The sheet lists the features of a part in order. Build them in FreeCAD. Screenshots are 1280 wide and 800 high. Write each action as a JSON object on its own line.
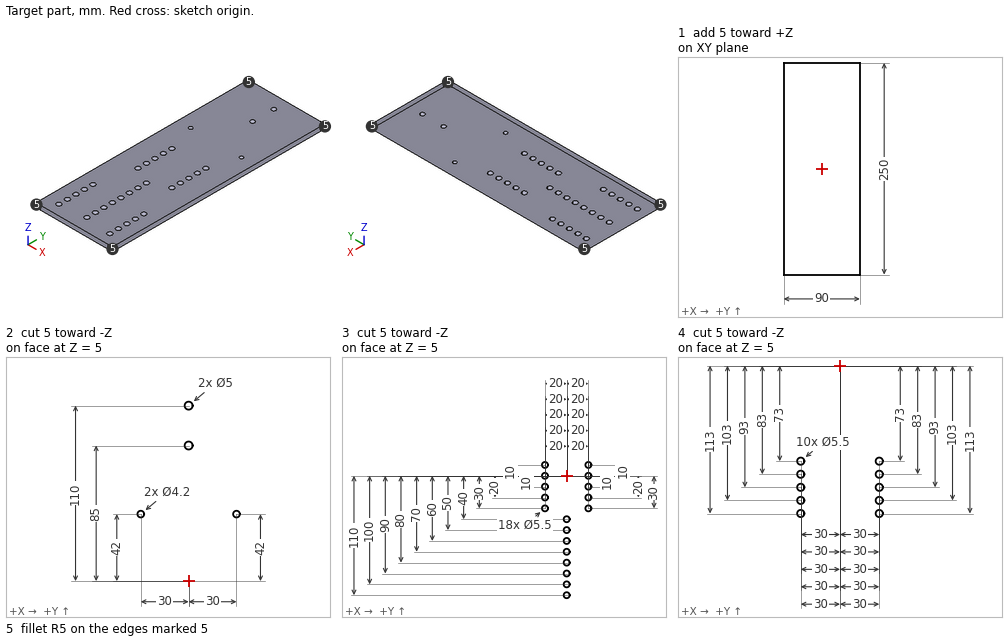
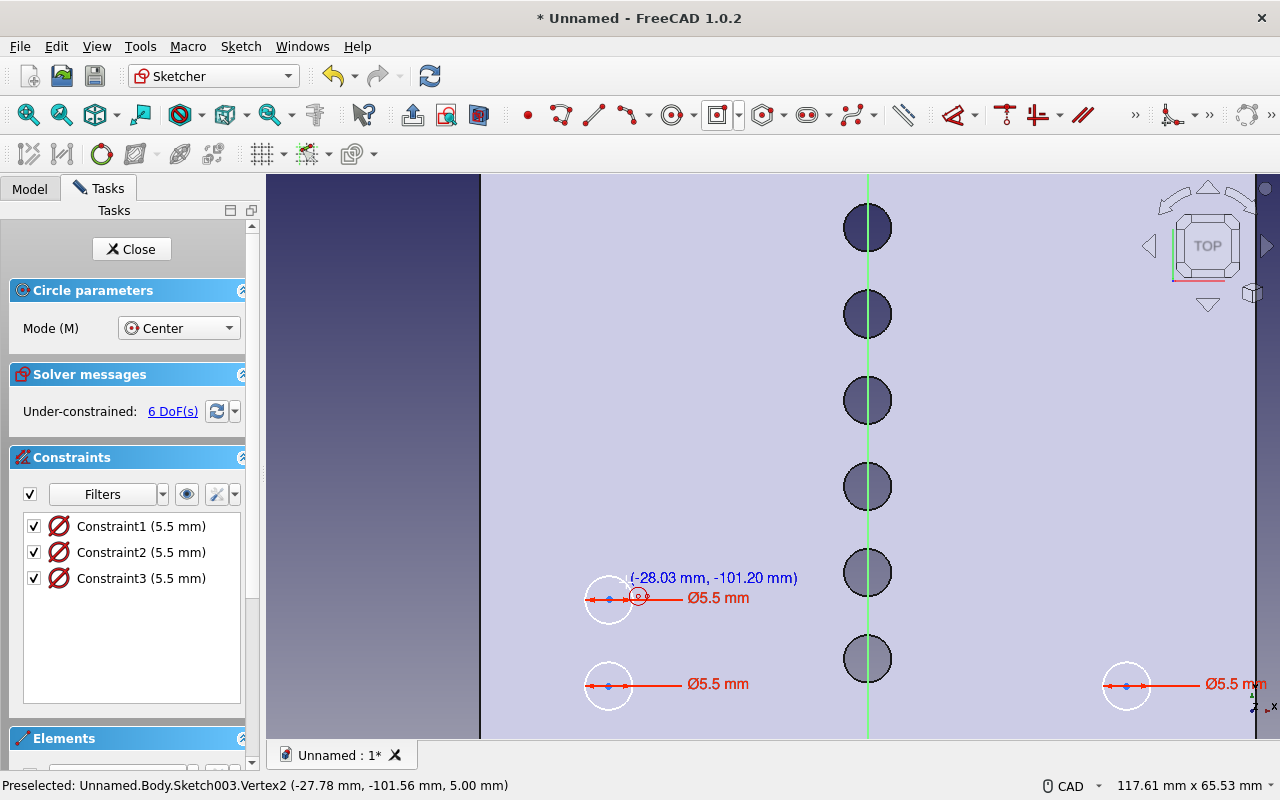
{"action": "scroll", "coordinate": [610, 600], "scroll_direction": "down", "scroll_amount": 5}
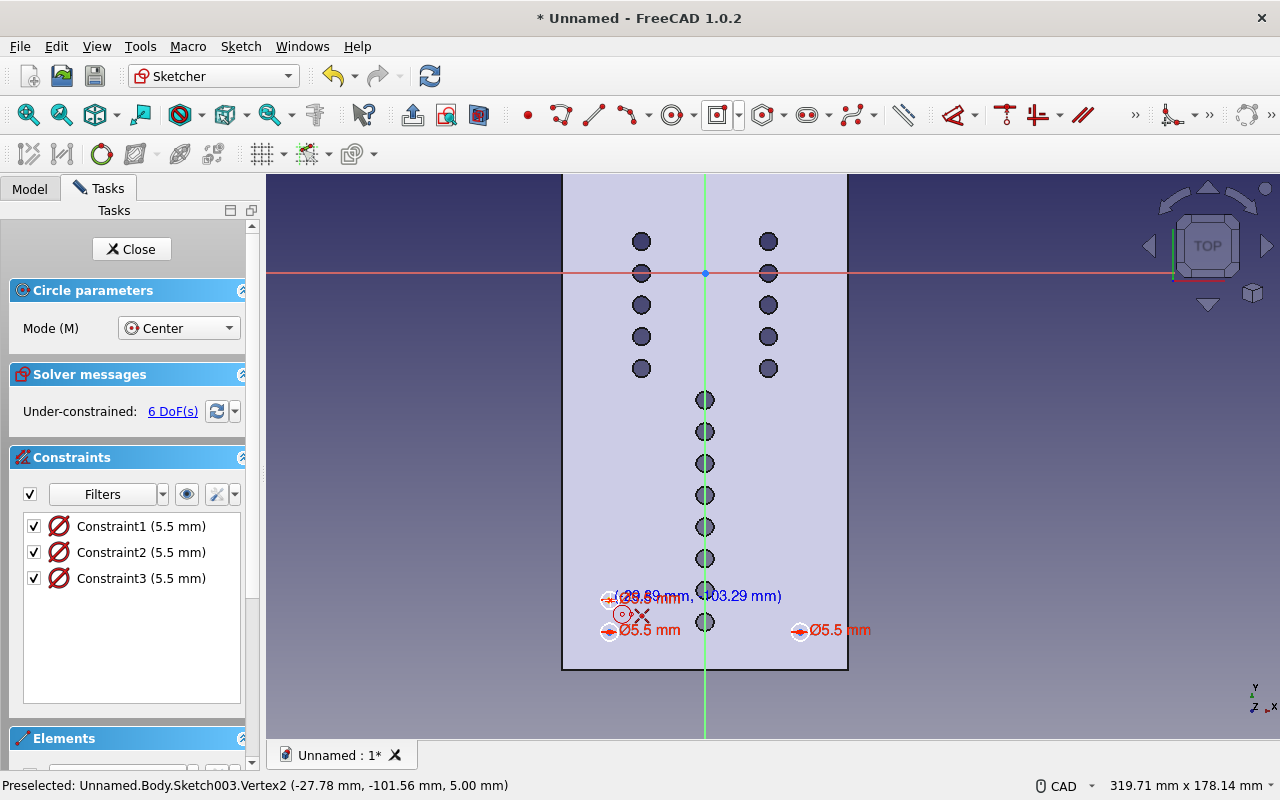
{"action": "scroll", "coordinate": [800, 600], "scroll_direction": "up", "scroll_amount": 5}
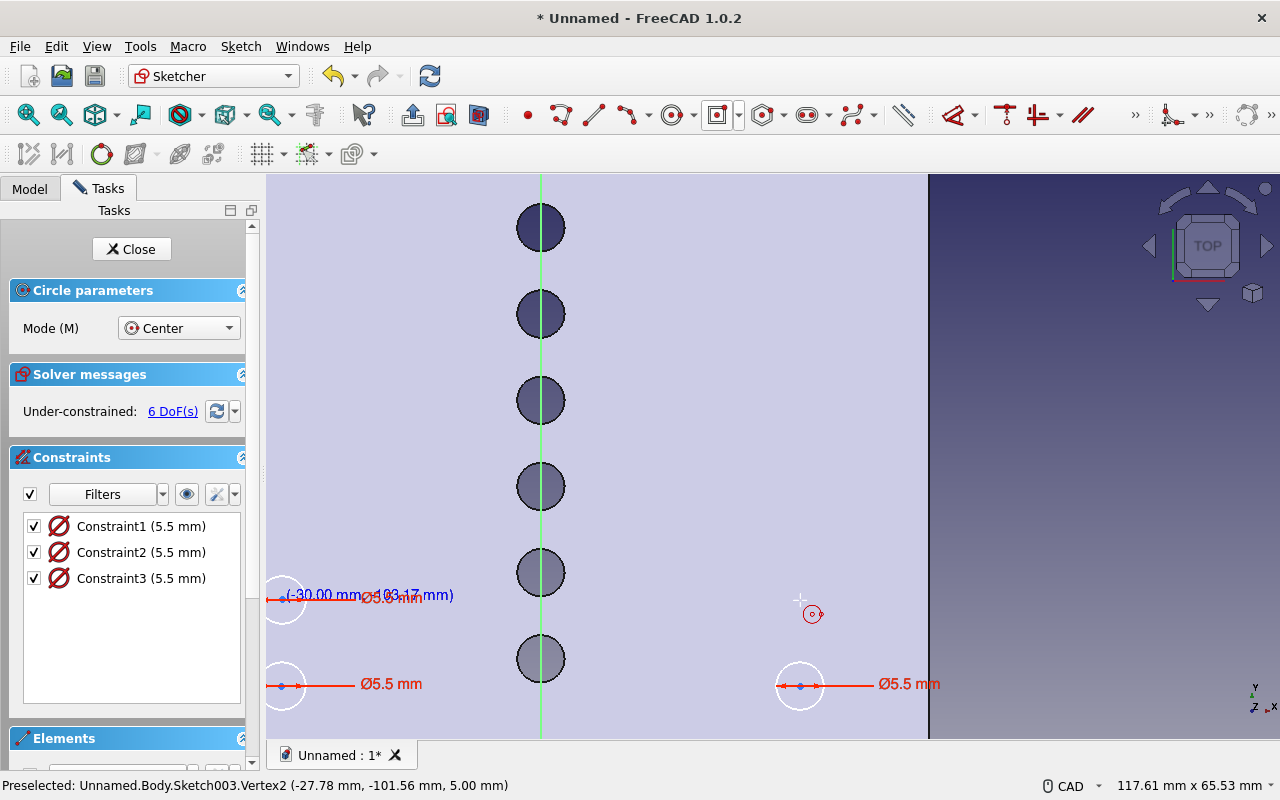
{"action": "left_click", "coordinate": [800, 599]}
{"action": "mouse_move", "coordinate": [816, 582]}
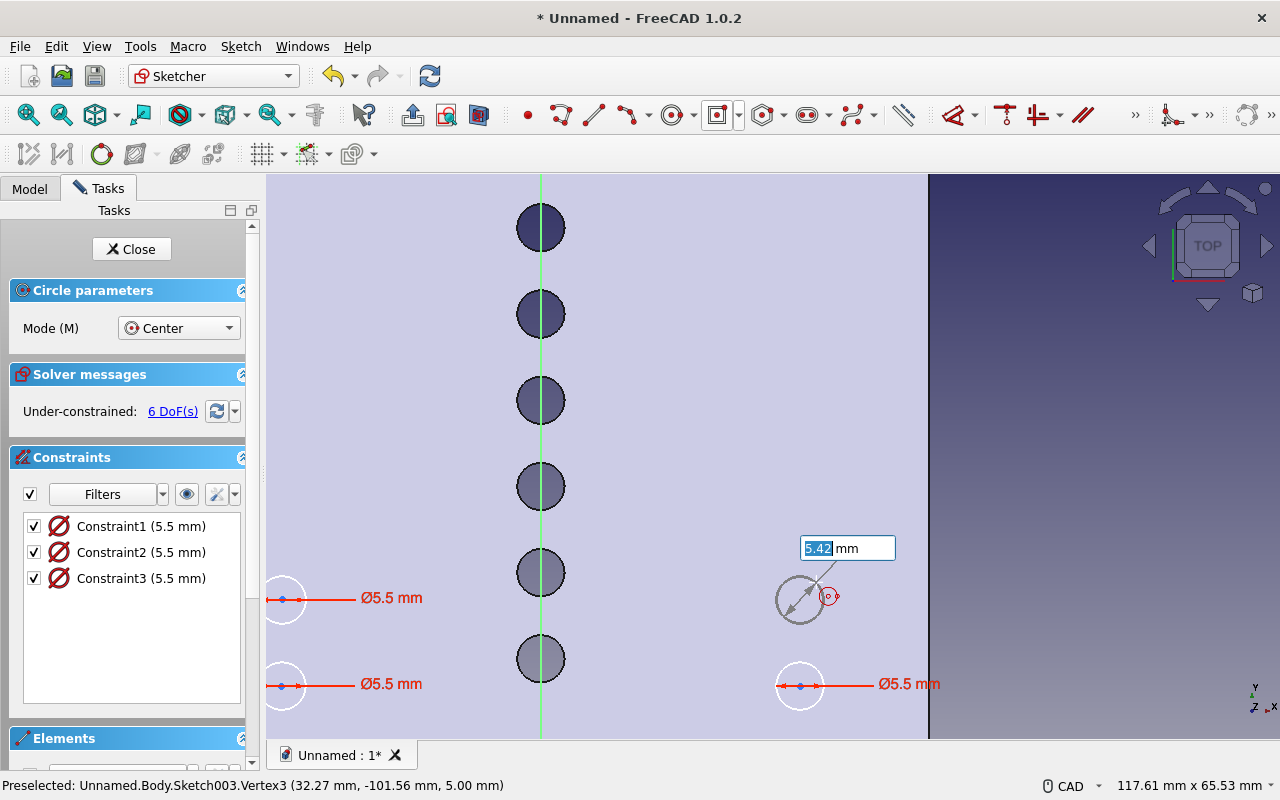
{"action": "type", "text": "5.5"}
{"action": "key", "text": "Return"}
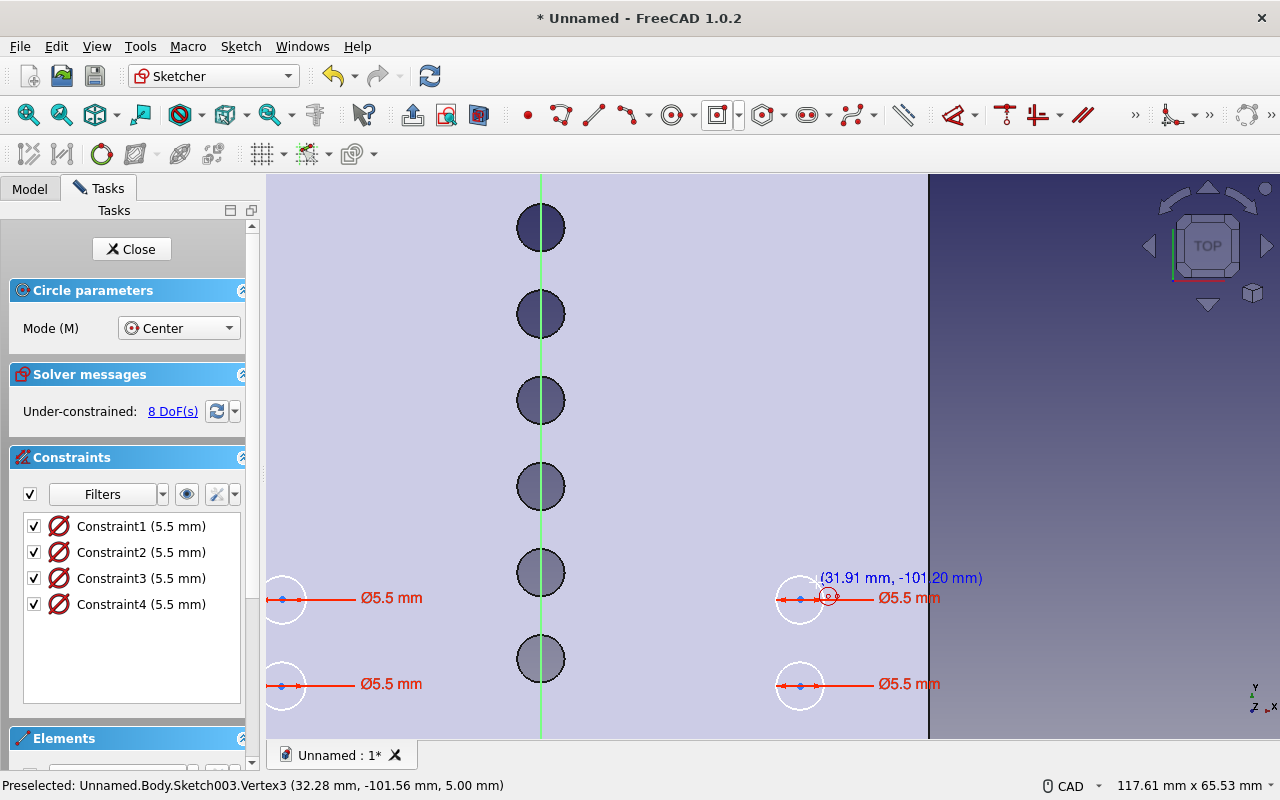
{"action": "scroll", "coordinate": [800, 600], "scroll_direction": "down", "scroll_amount": 5}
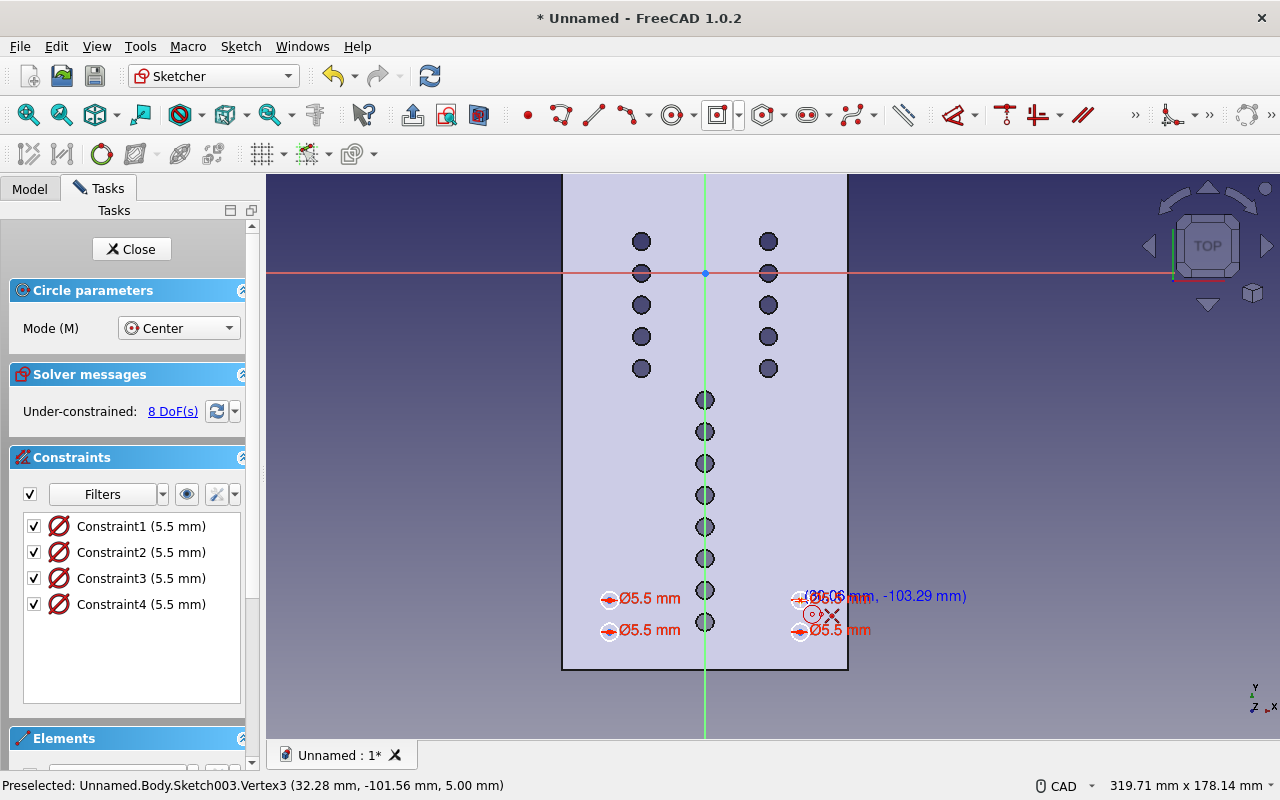
{"action": "scroll", "coordinate": [610, 568], "scroll_direction": "up", "scroll_amount": 5}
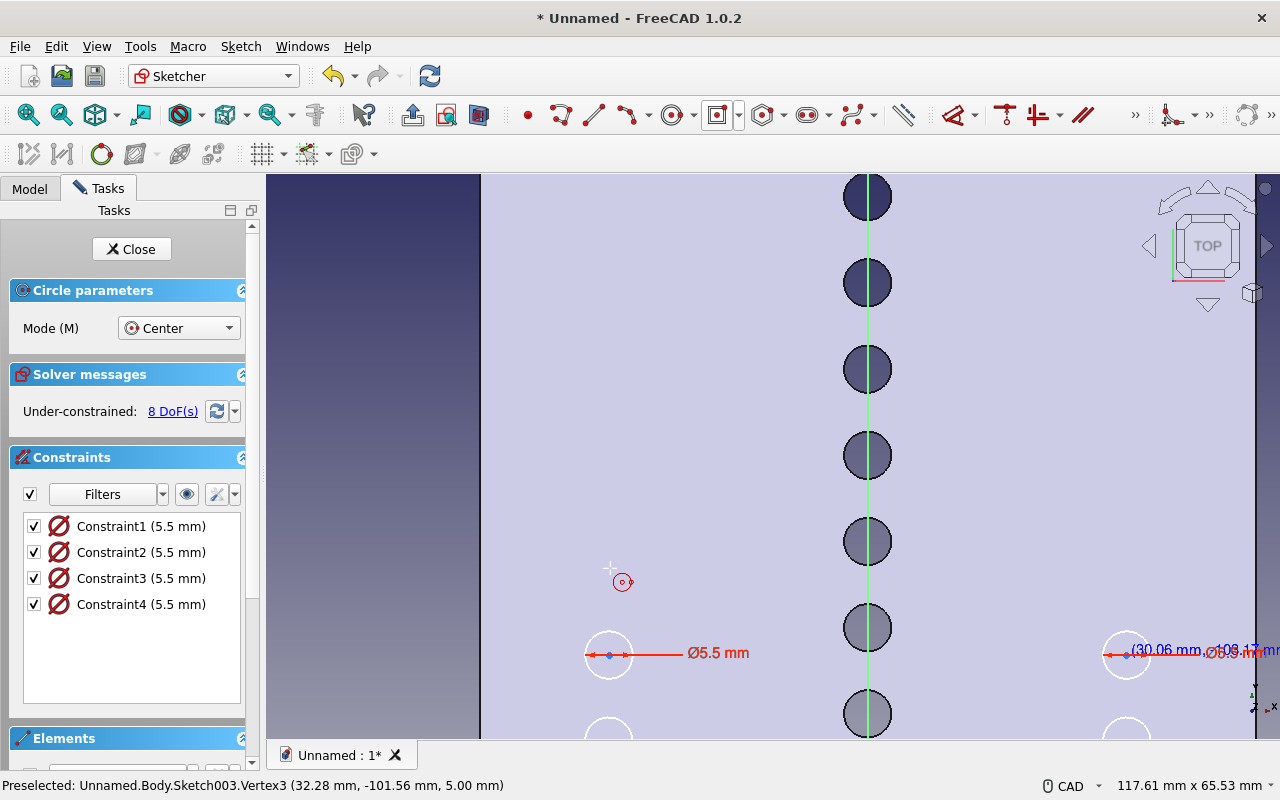
{"action": "left_click", "coordinate": [609, 567]}
{"action": "mouse_move", "coordinate": [626, 551]}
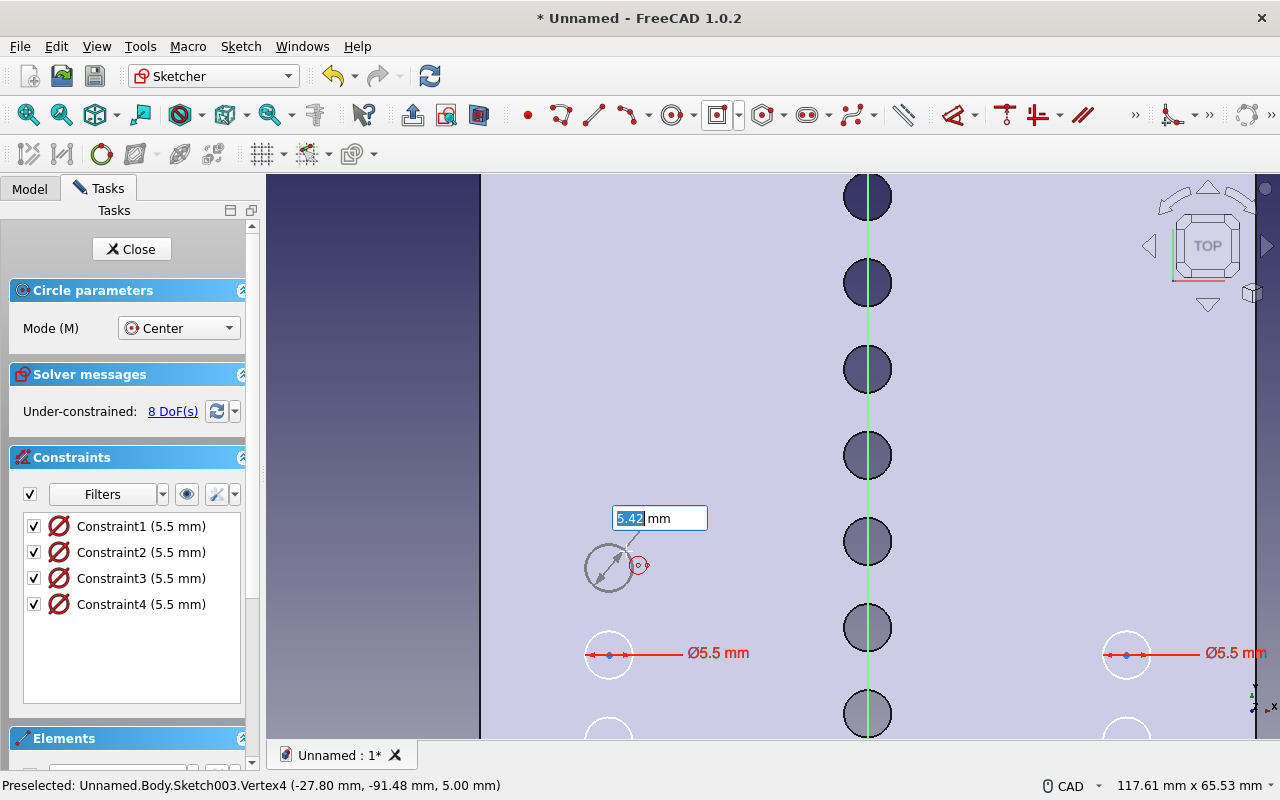
{"action": "type", "text": "5.5"}
{"action": "key", "text": "Return"}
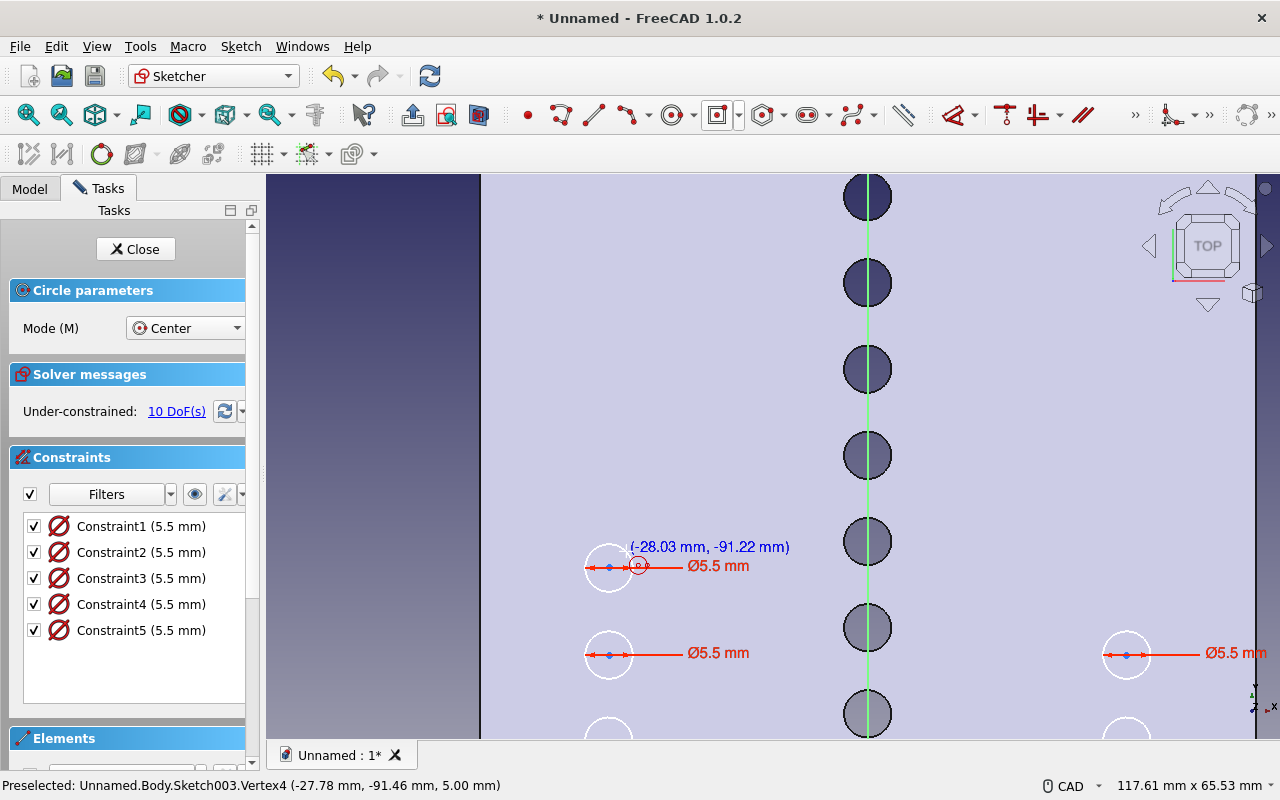
{"action": "scroll", "coordinate": [610, 568], "scroll_direction": "down", "scroll_amount": 5}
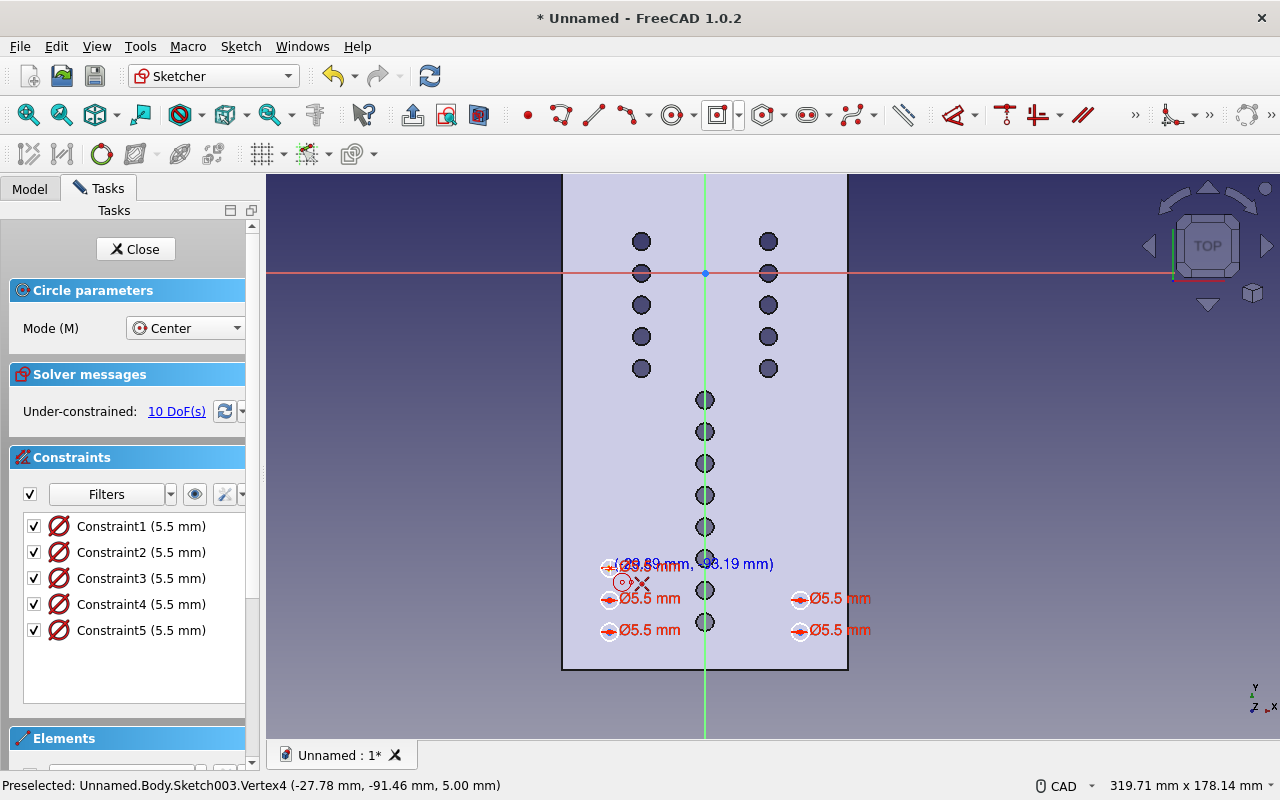
{"action": "scroll", "coordinate": [800, 568], "scroll_direction": "up", "scroll_amount": 5}